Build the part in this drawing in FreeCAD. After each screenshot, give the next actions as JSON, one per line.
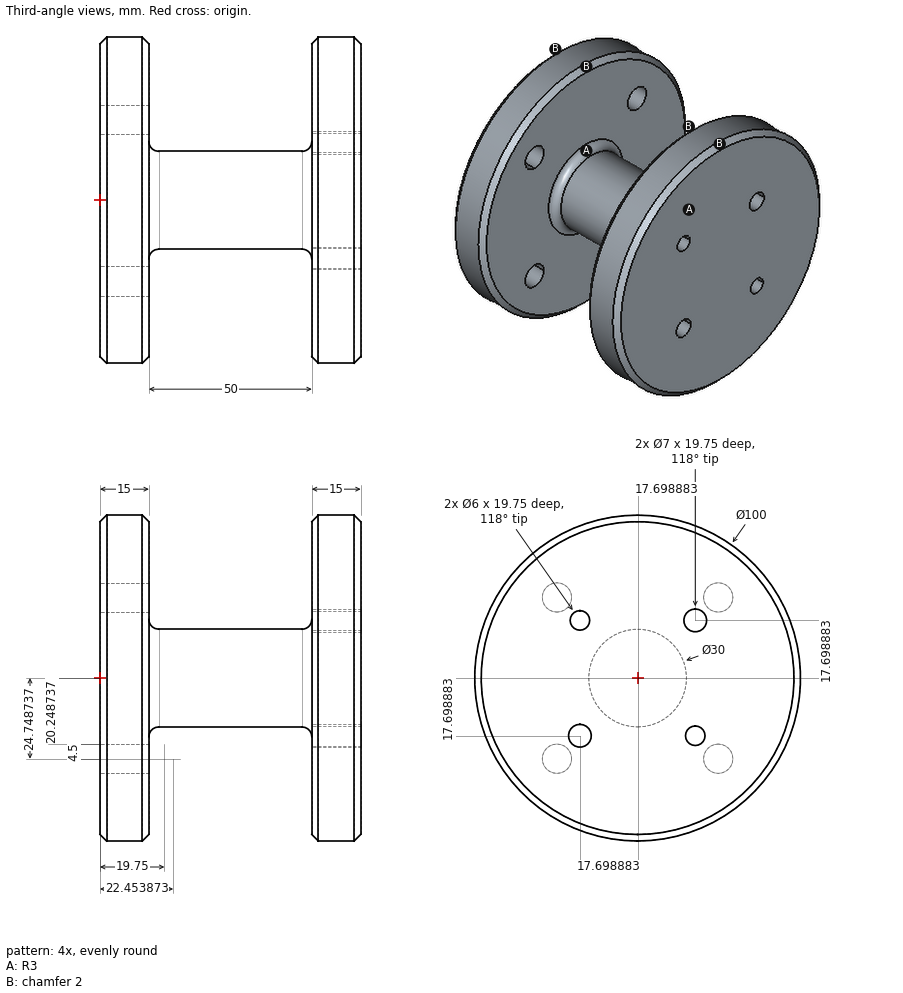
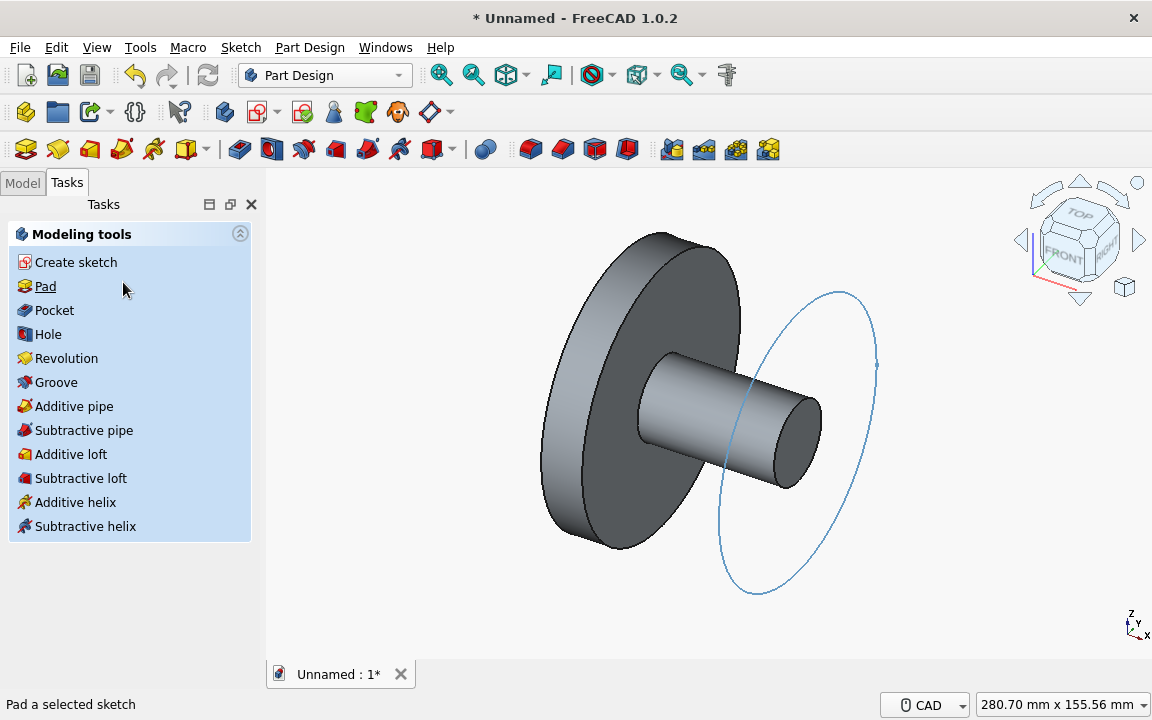
{"action": "left_click", "coordinate": [26, 150]}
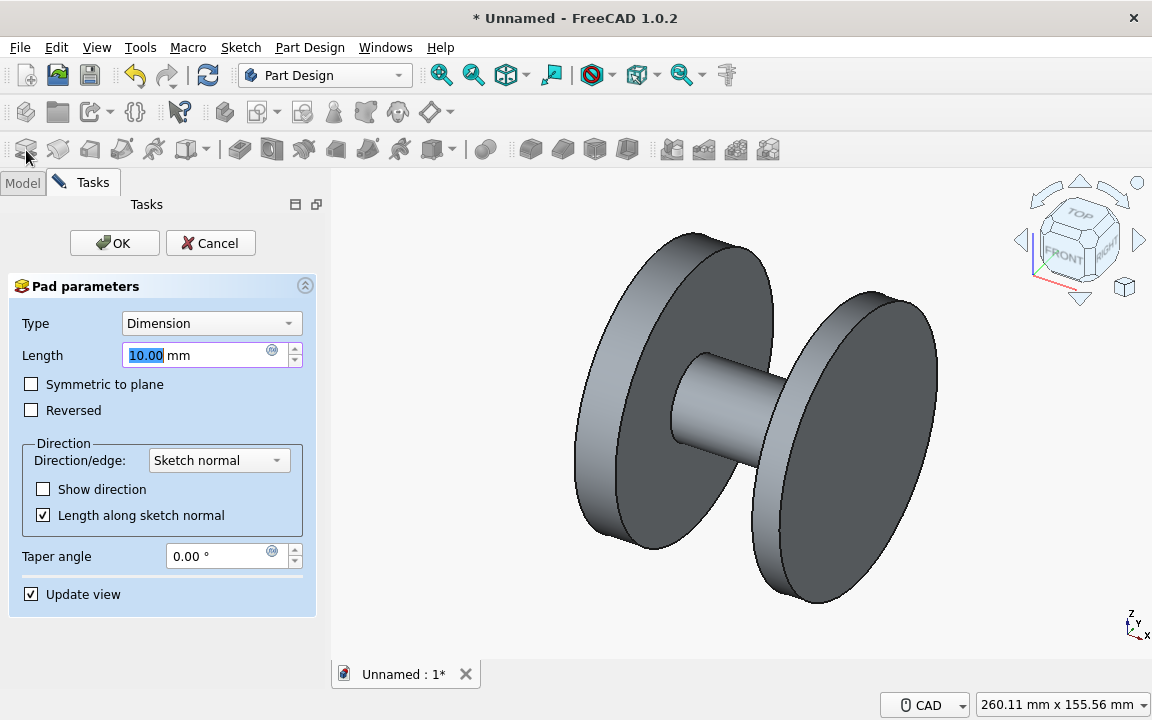
{"action": "type", "text": "15"}
{"action": "key", "text": "Tab"}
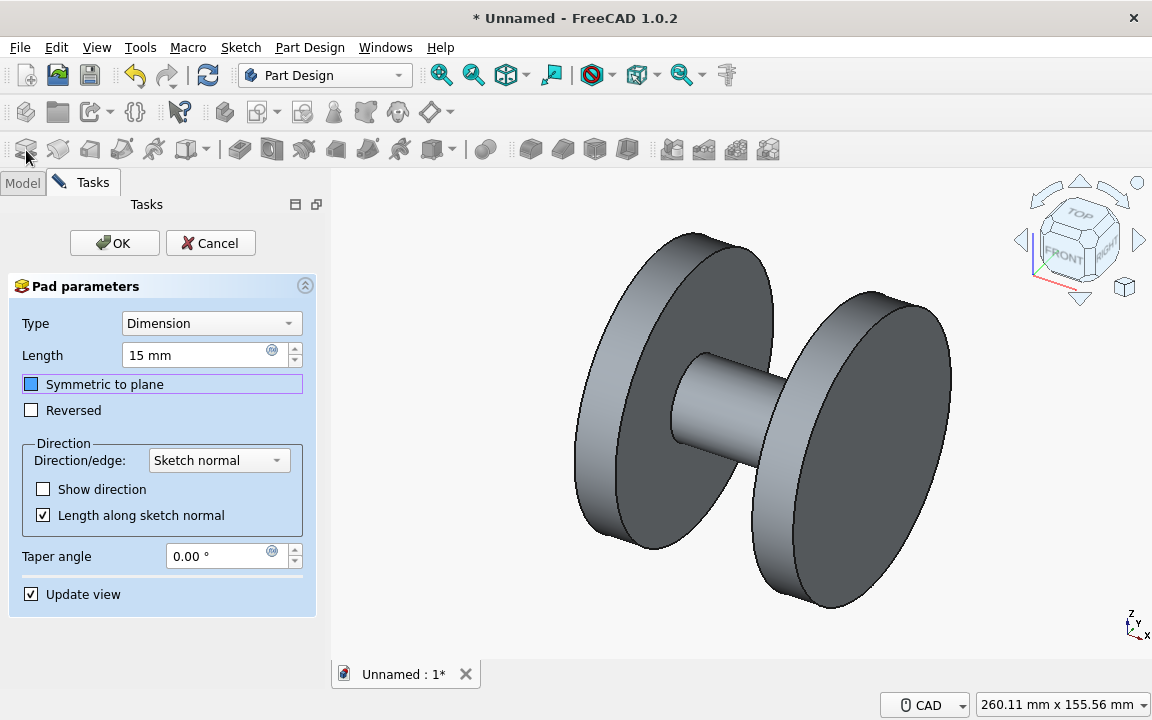
{"action": "left_click", "coordinate": [115, 243]}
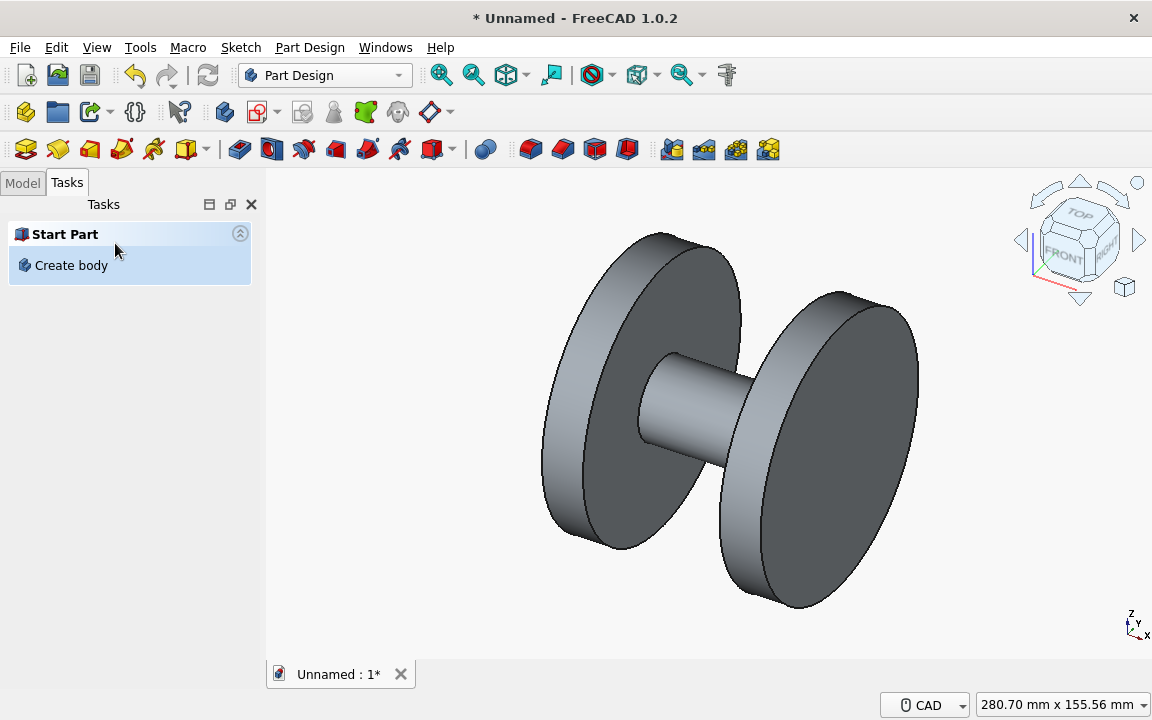
{"action": "left_click", "coordinate": [442, 76]}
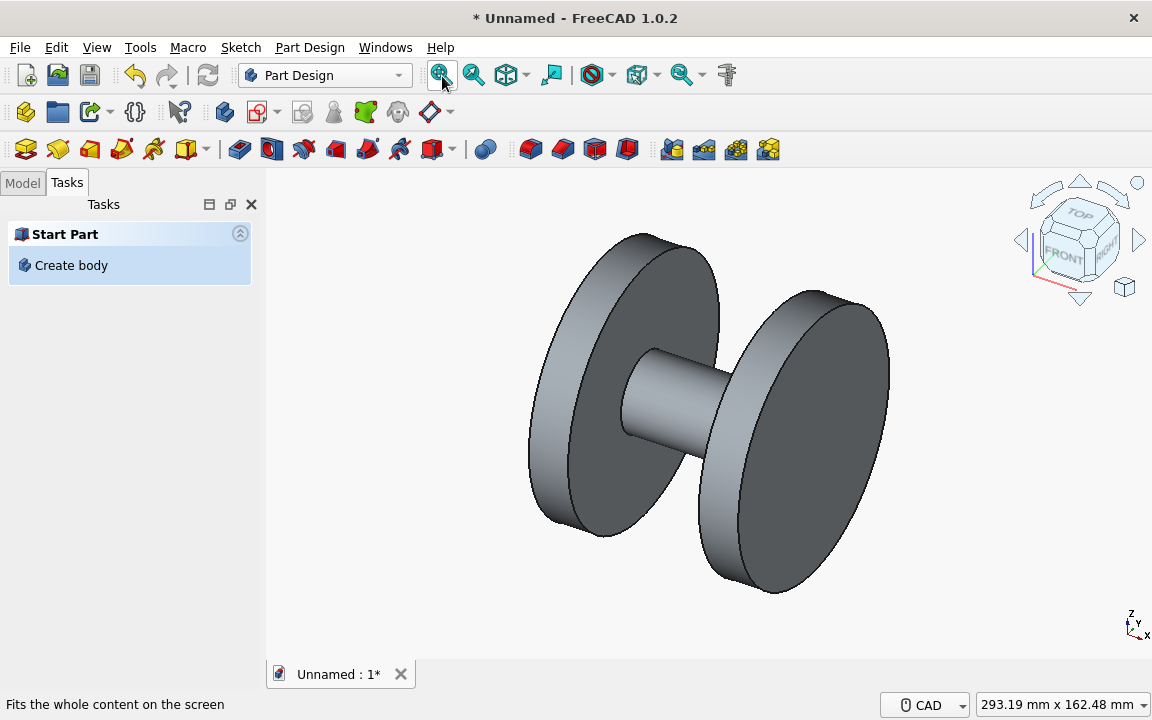
{"action": "left_click", "coordinate": [814, 447]}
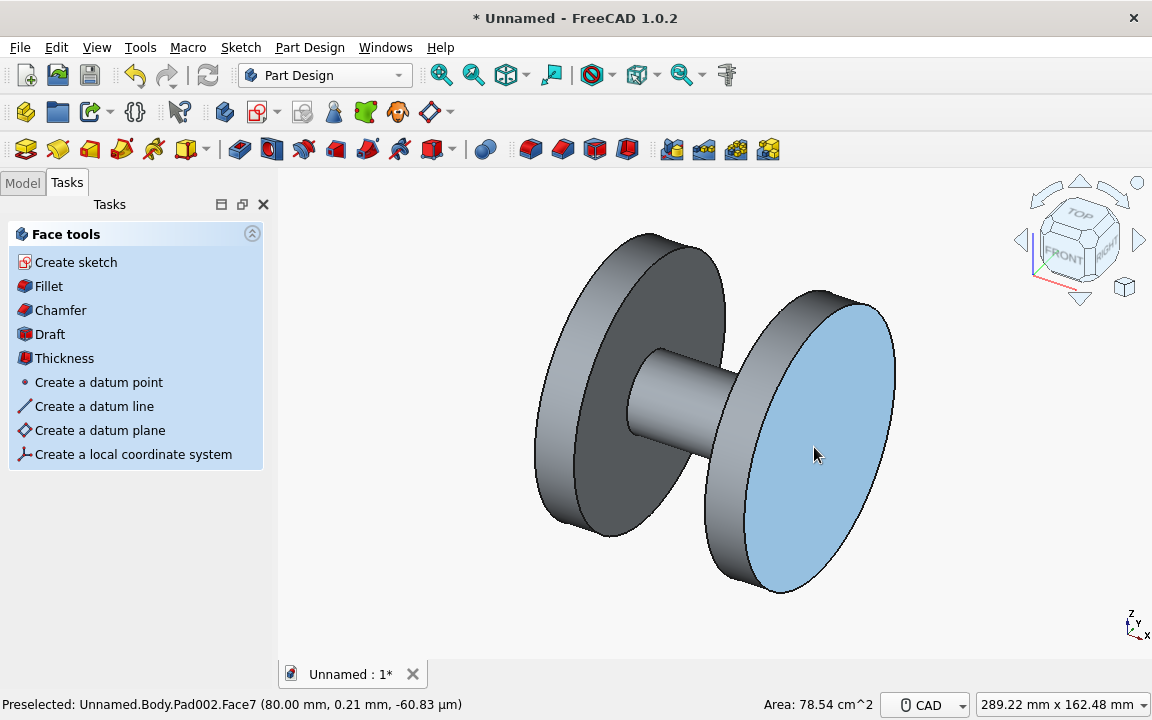
{"action": "left_click", "coordinate": [258, 112]}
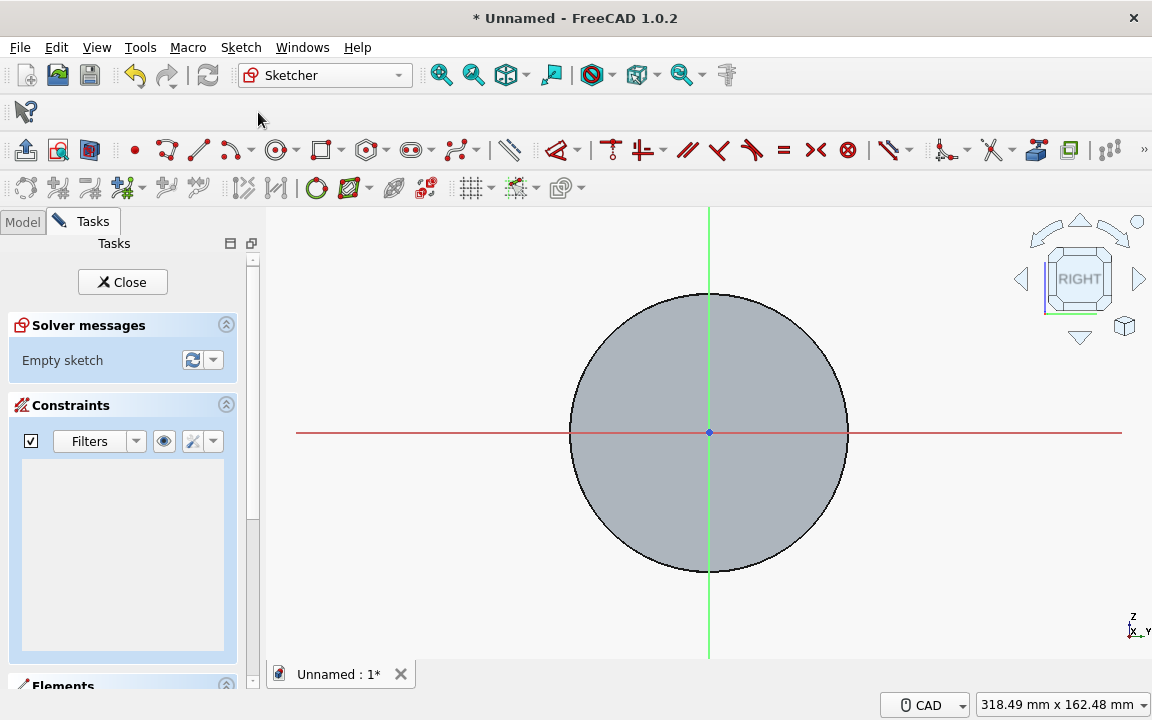
{"action": "scroll", "coordinate": [765, 433], "scroll_direction": "up", "scroll_amount": 4}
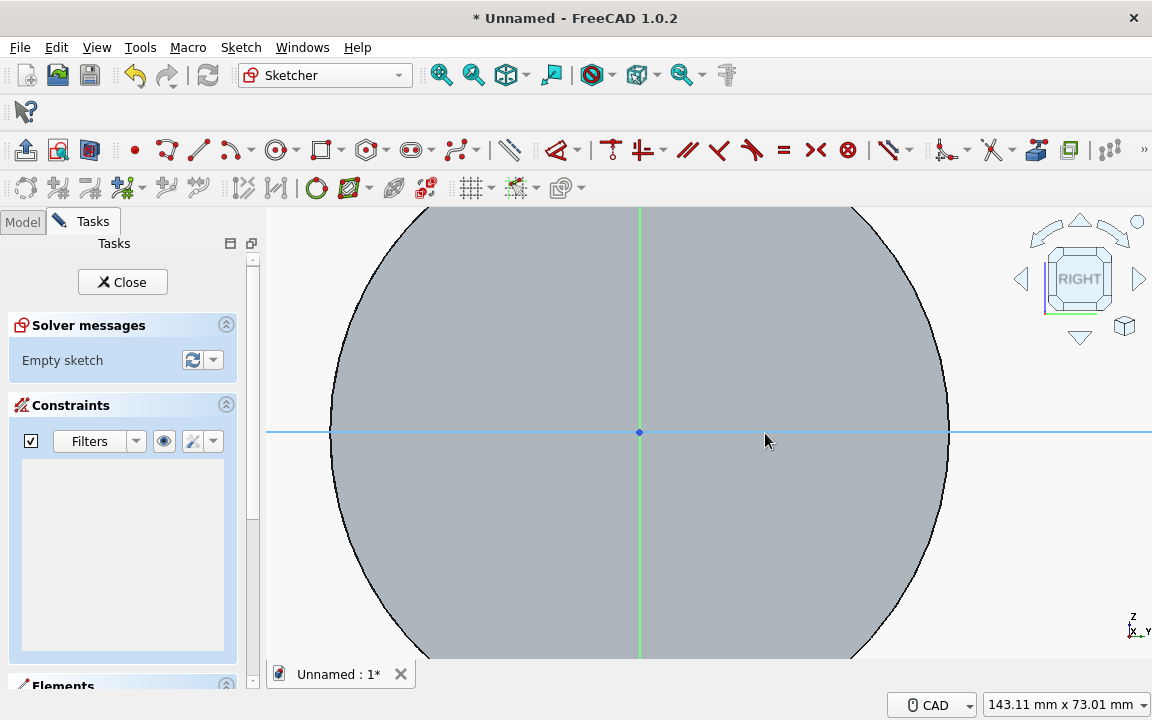
{"action": "key", "text": "g c"}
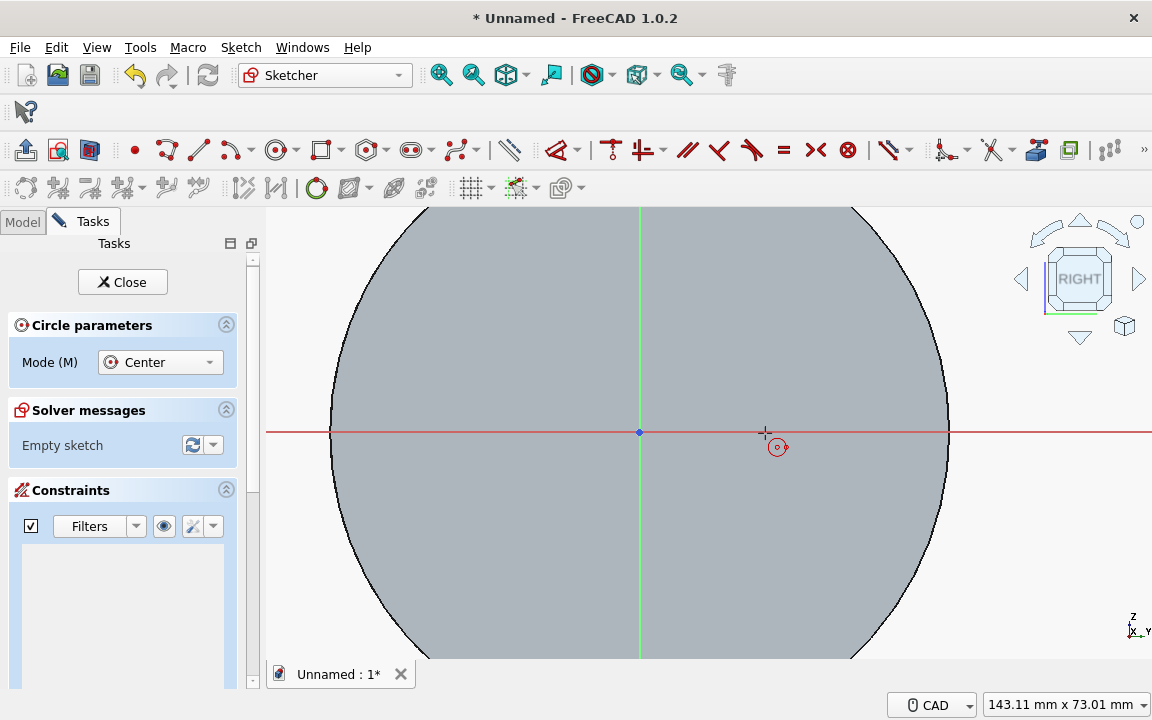
{"action": "left_click", "coordinate": [749, 323]}
{"action": "left_click", "coordinate": [765, 307]}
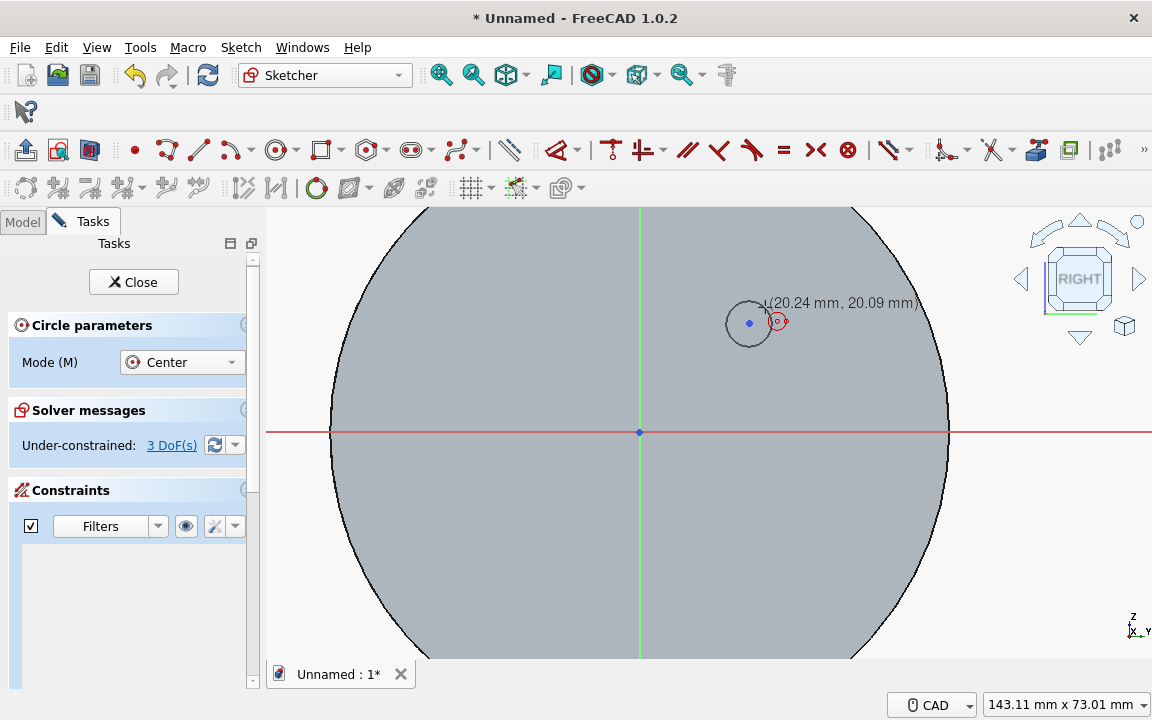
{"action": "left_click", "coordinate": [530, 542]}
{"action": "left_click", "coordinate": [545, 527]}
{"action": "key", "text": "Escape"}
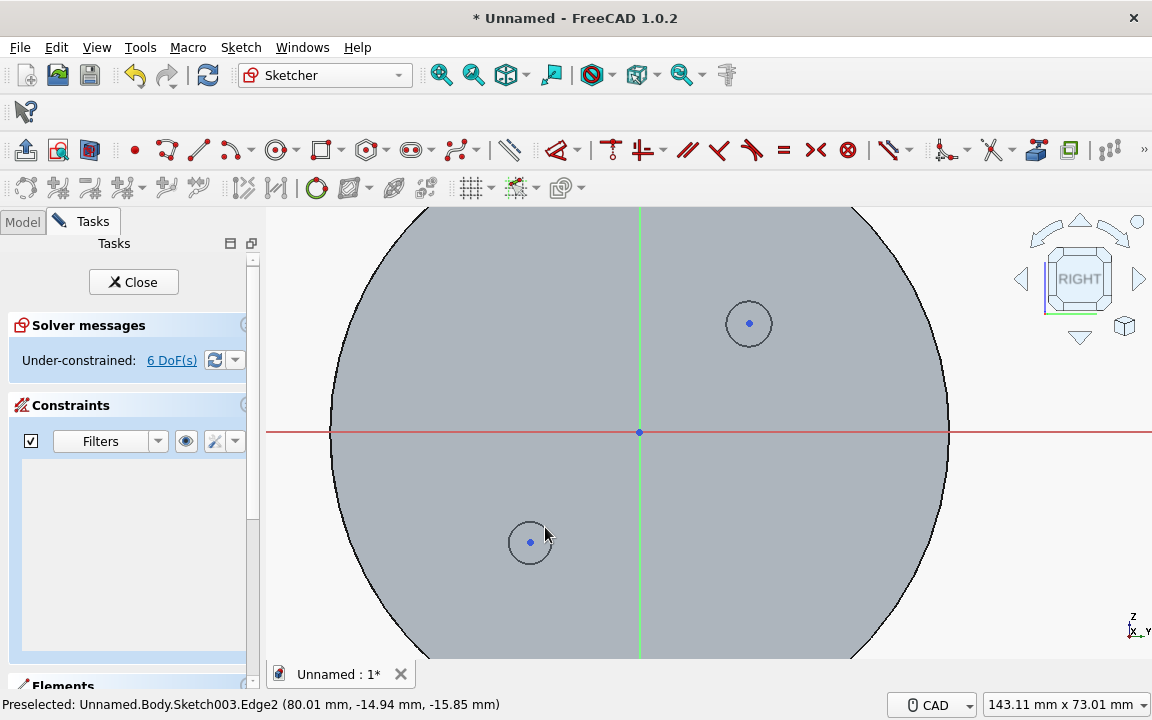
{"action": "left_click", "coordinate": [765, 308]}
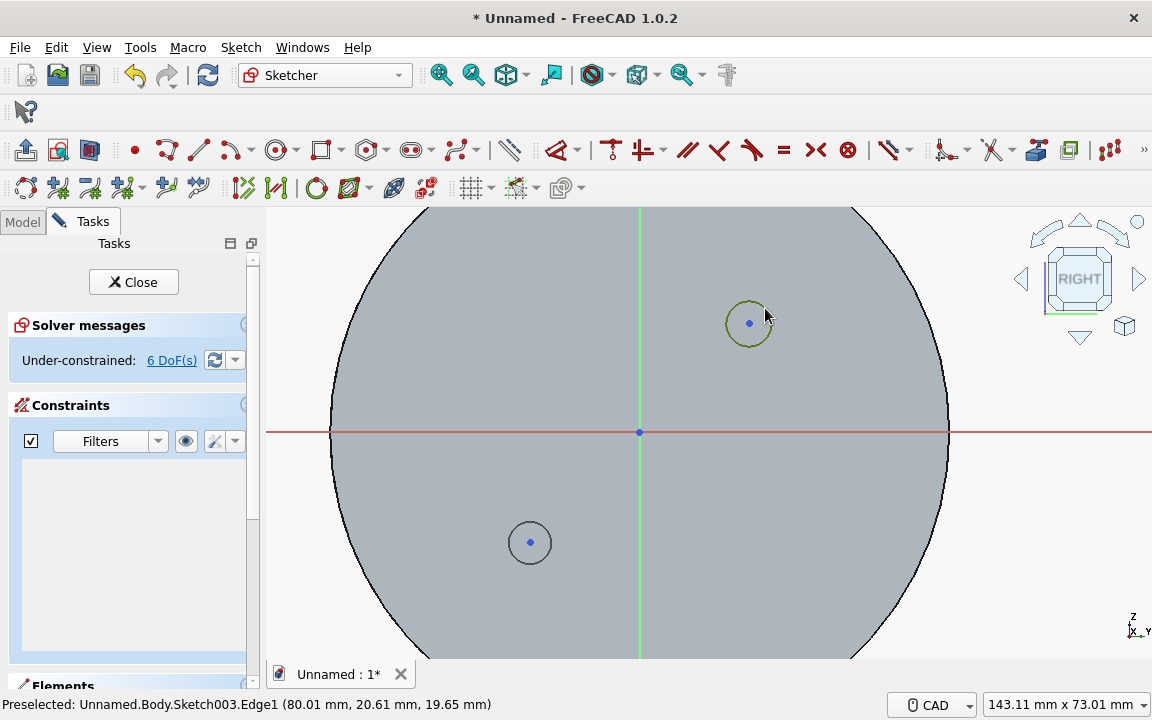
{"action": "left_click", "coordinate": [545, 528]}